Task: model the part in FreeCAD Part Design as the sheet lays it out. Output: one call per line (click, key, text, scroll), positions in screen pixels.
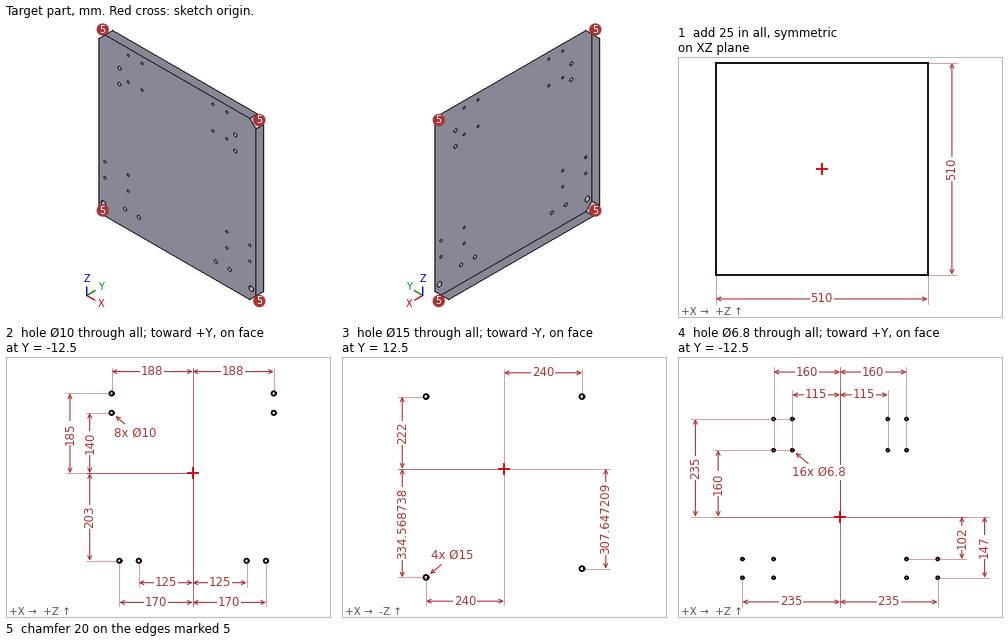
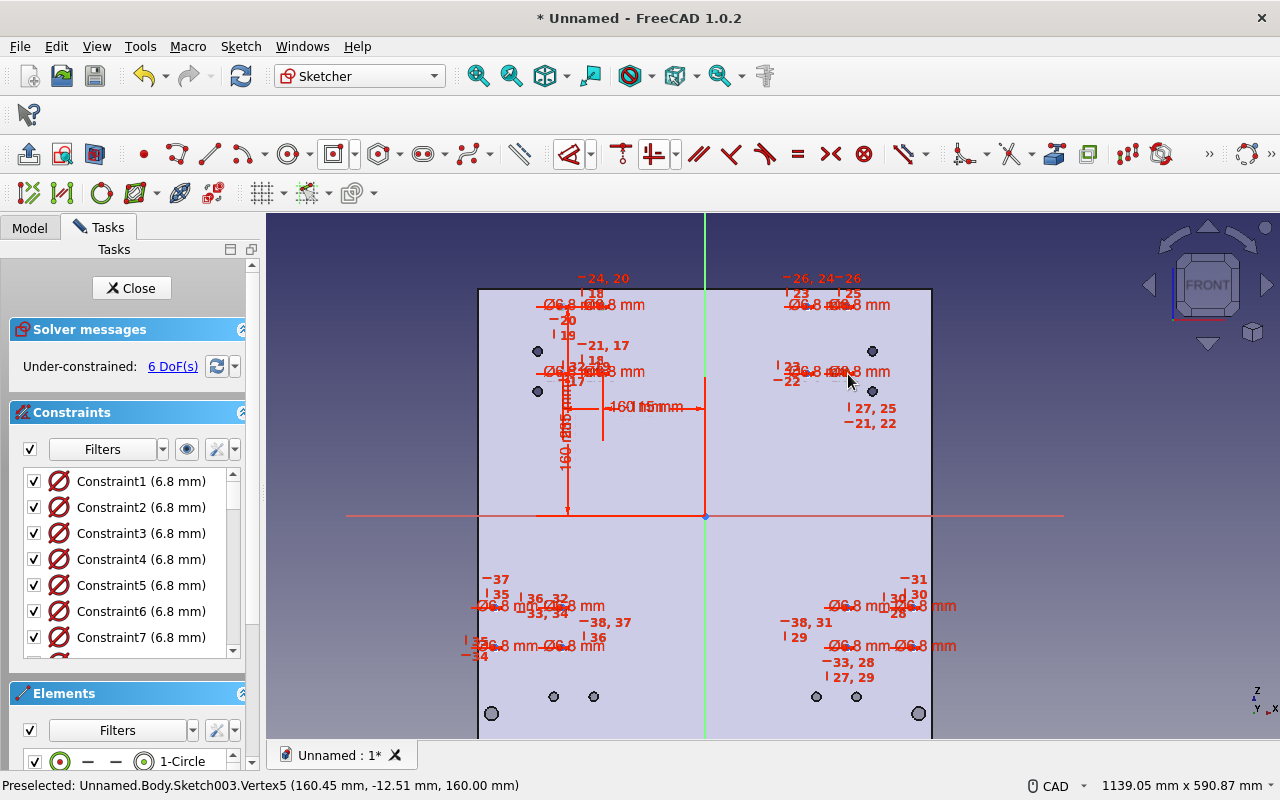
key(l)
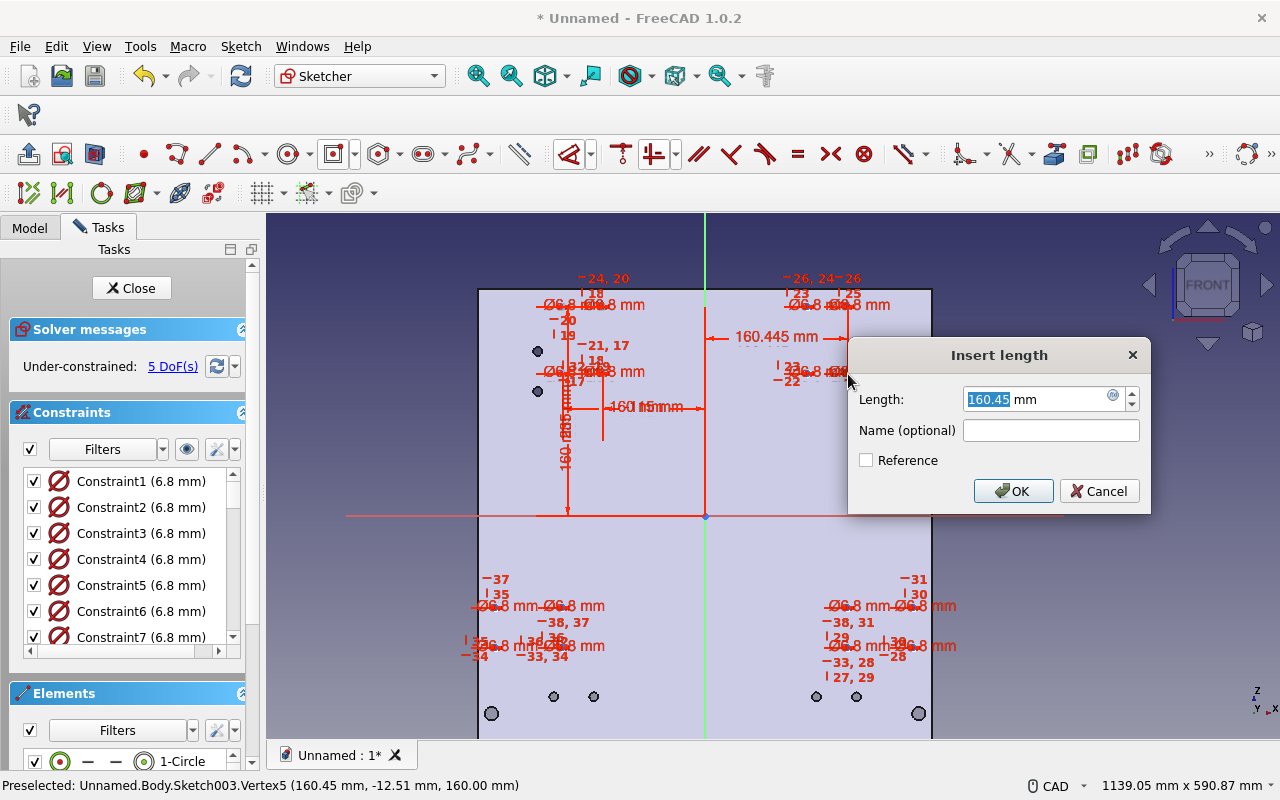
text(160)
key(Return)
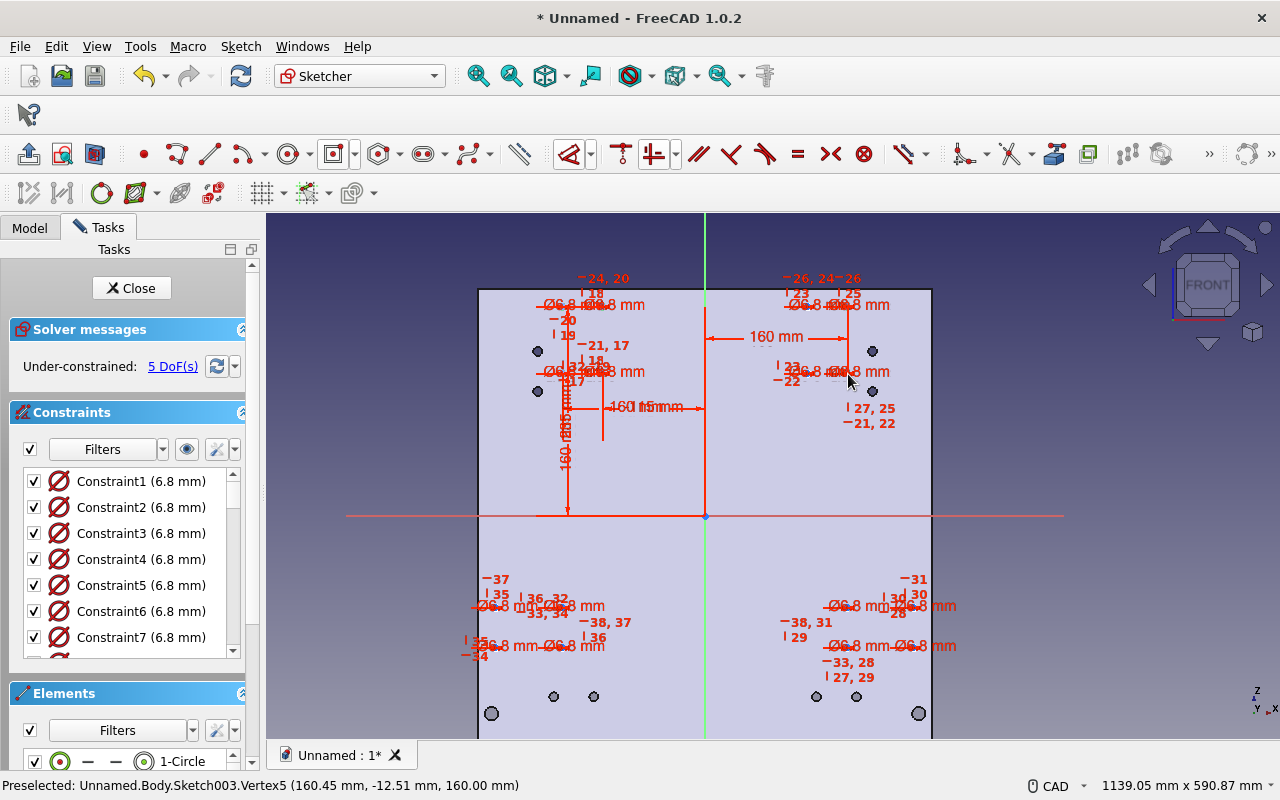
click(808, 374)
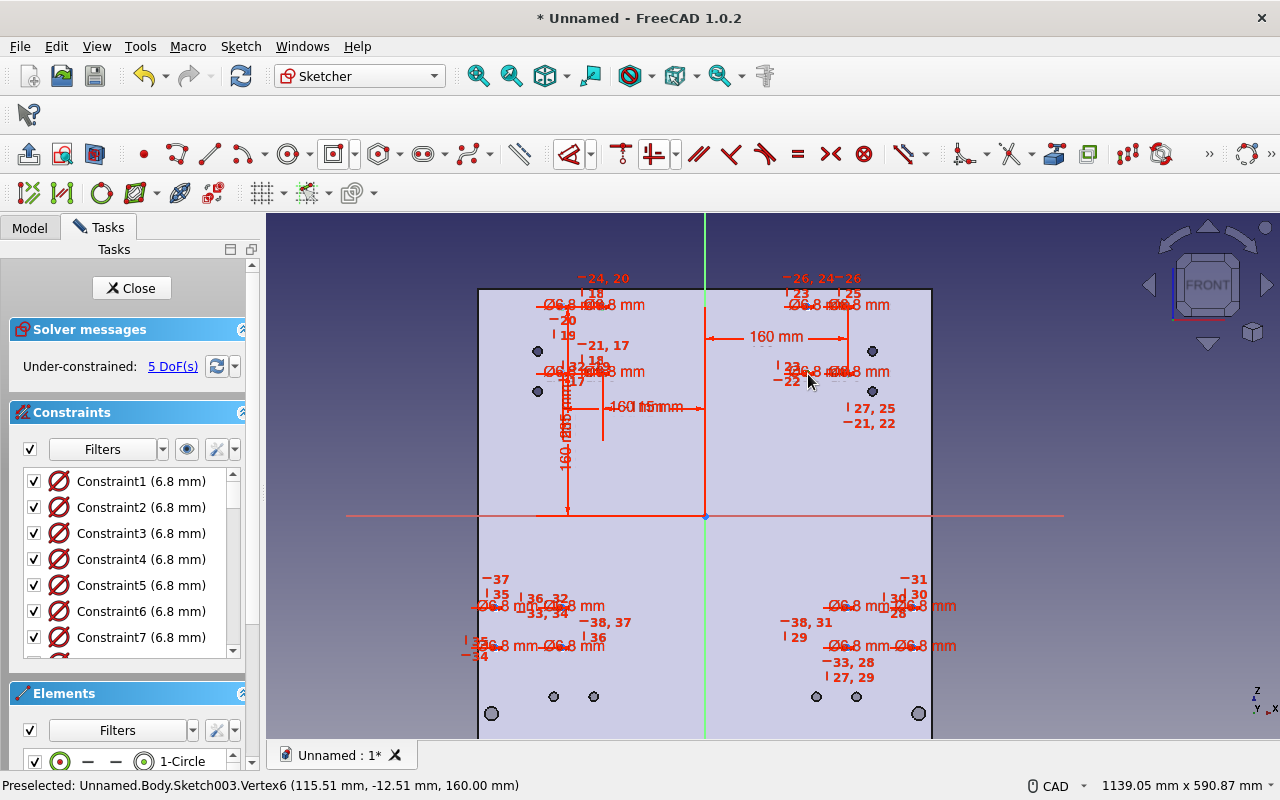
click(590, 154)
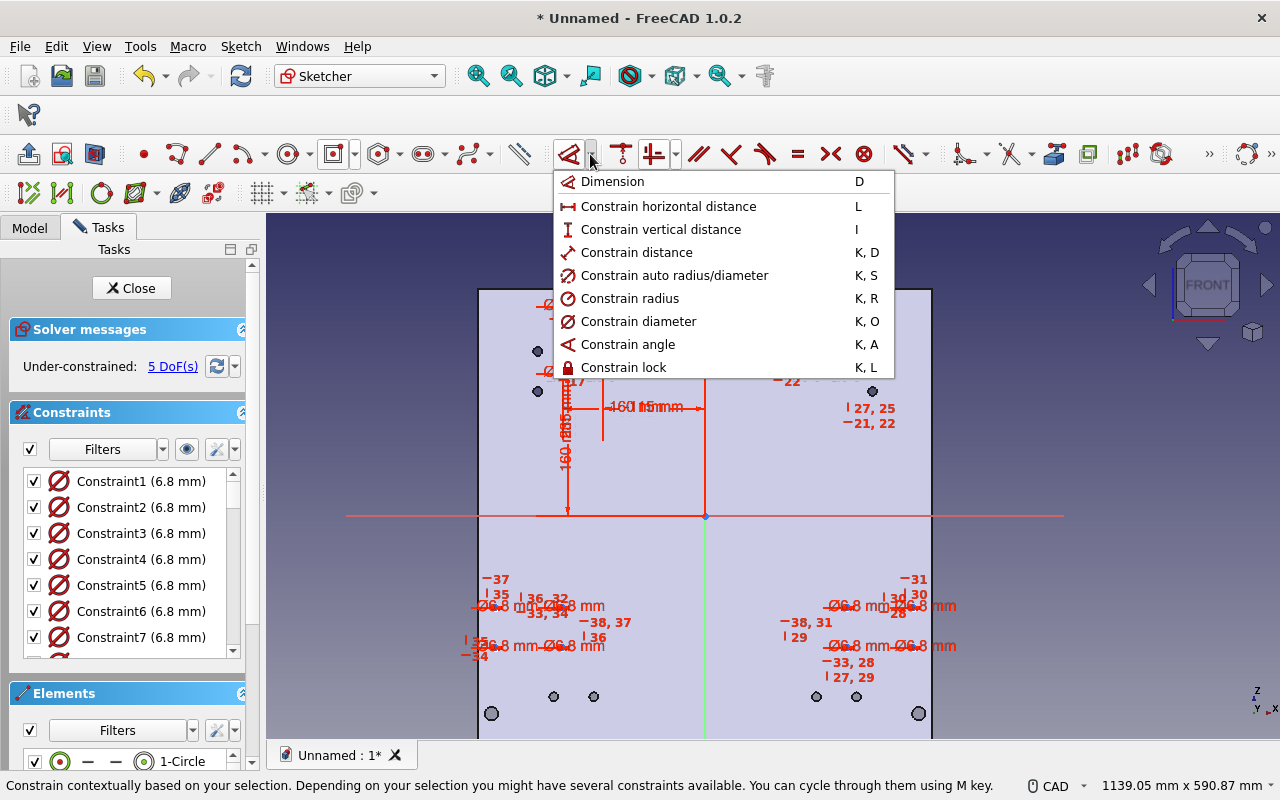
click(724, 206)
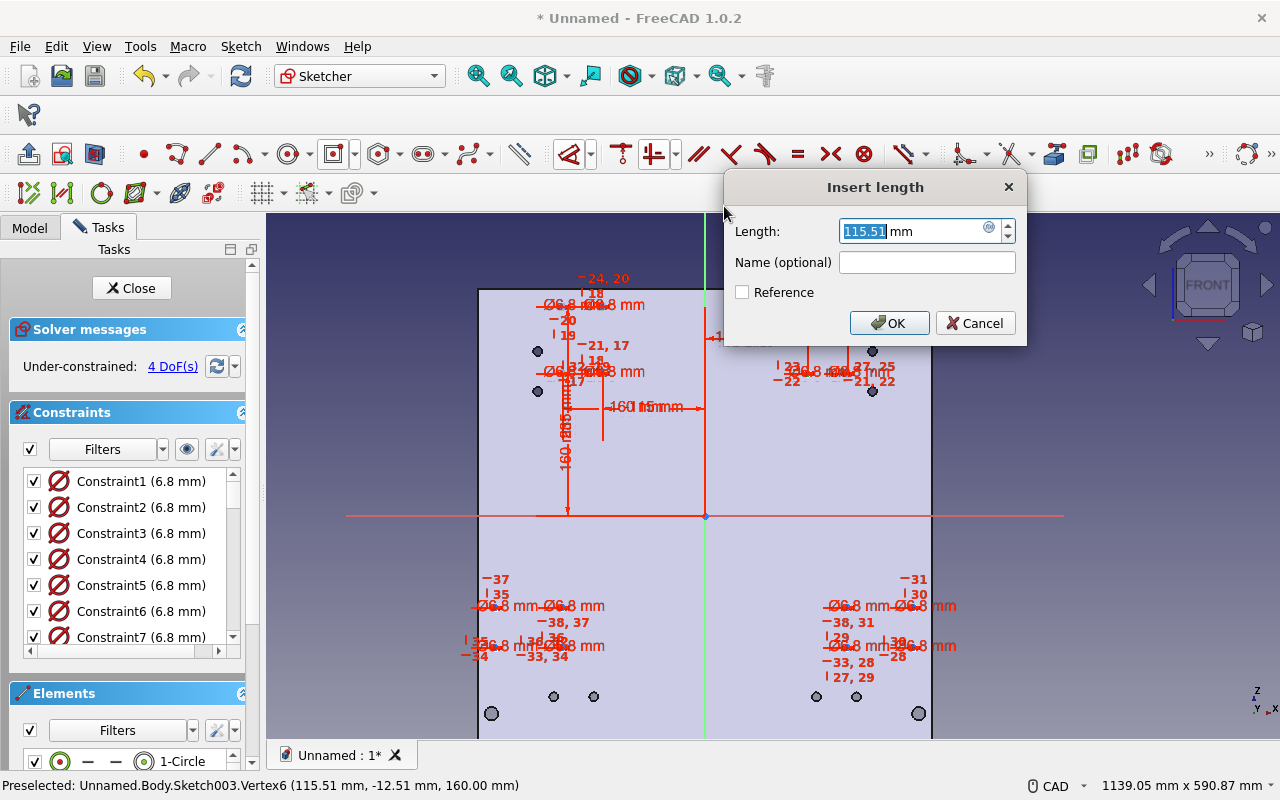
text(115)
key(Return)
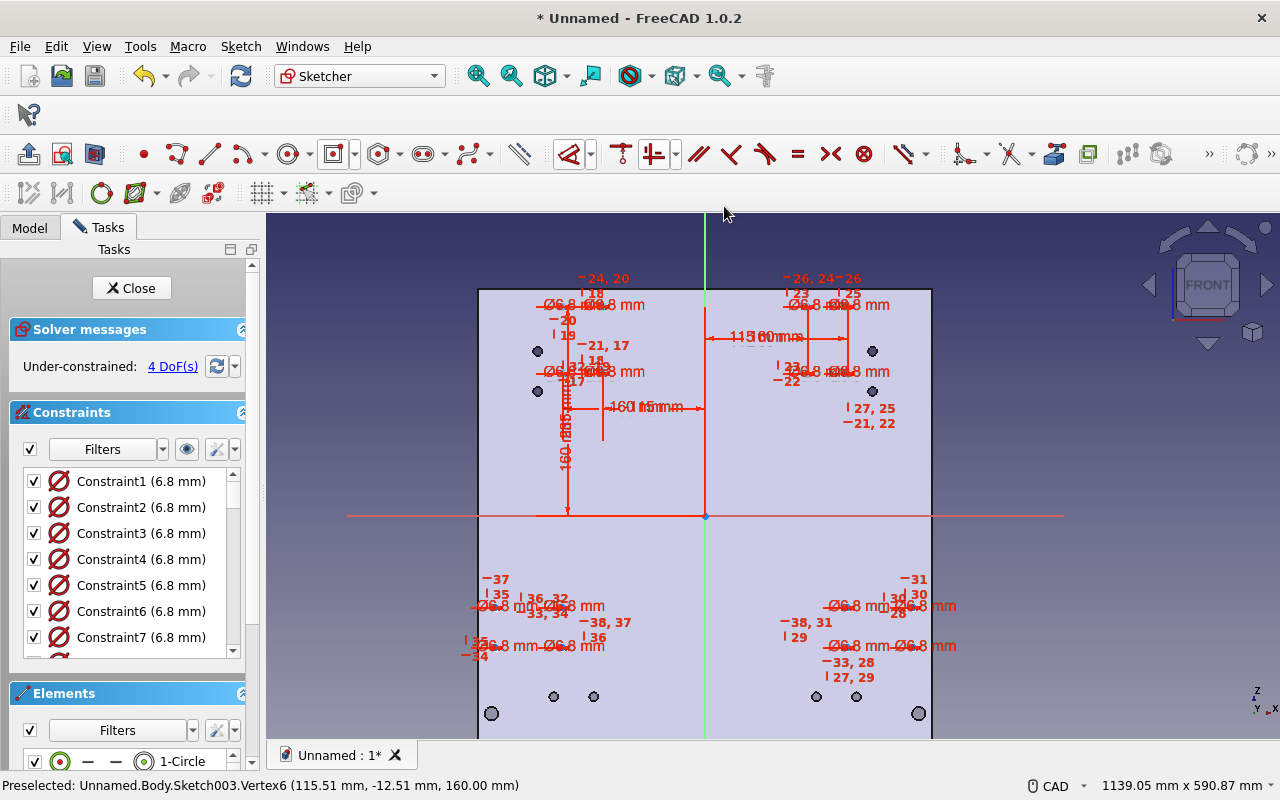
click(914, 648)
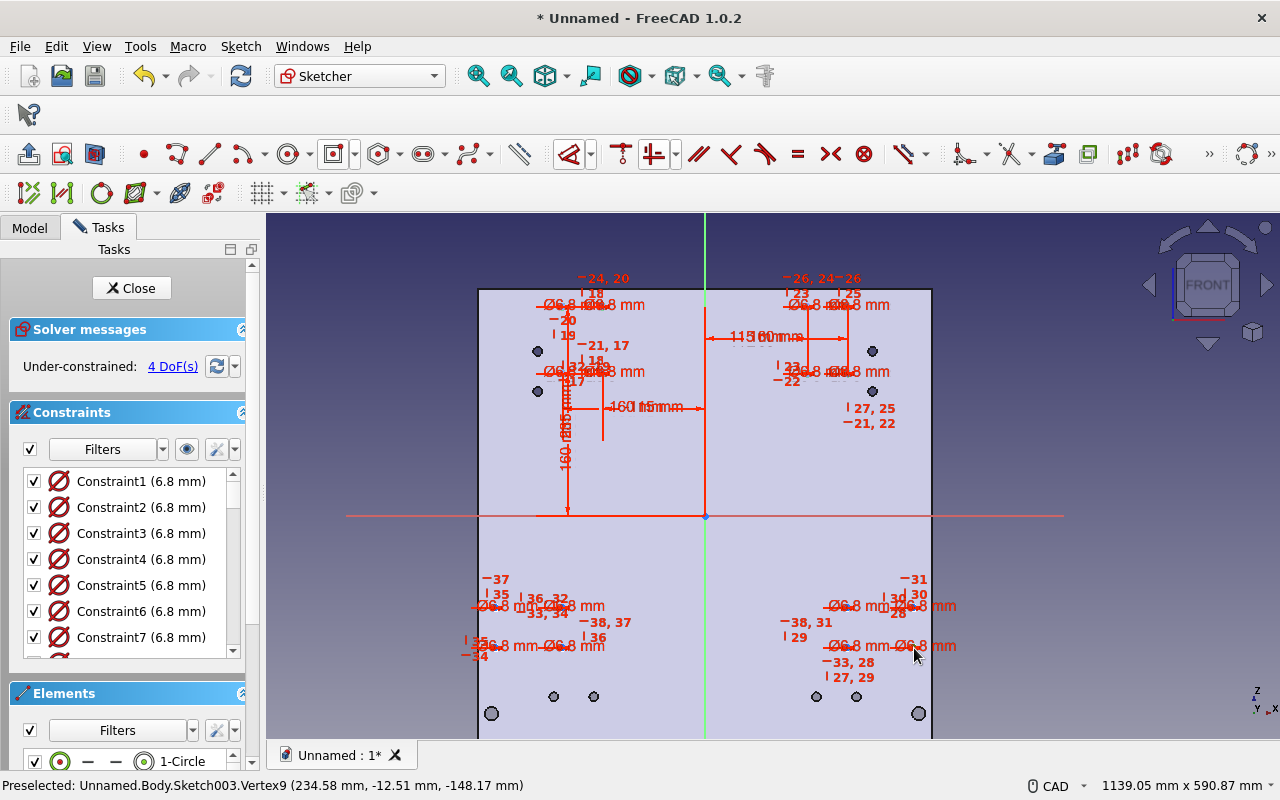
click(590, 154)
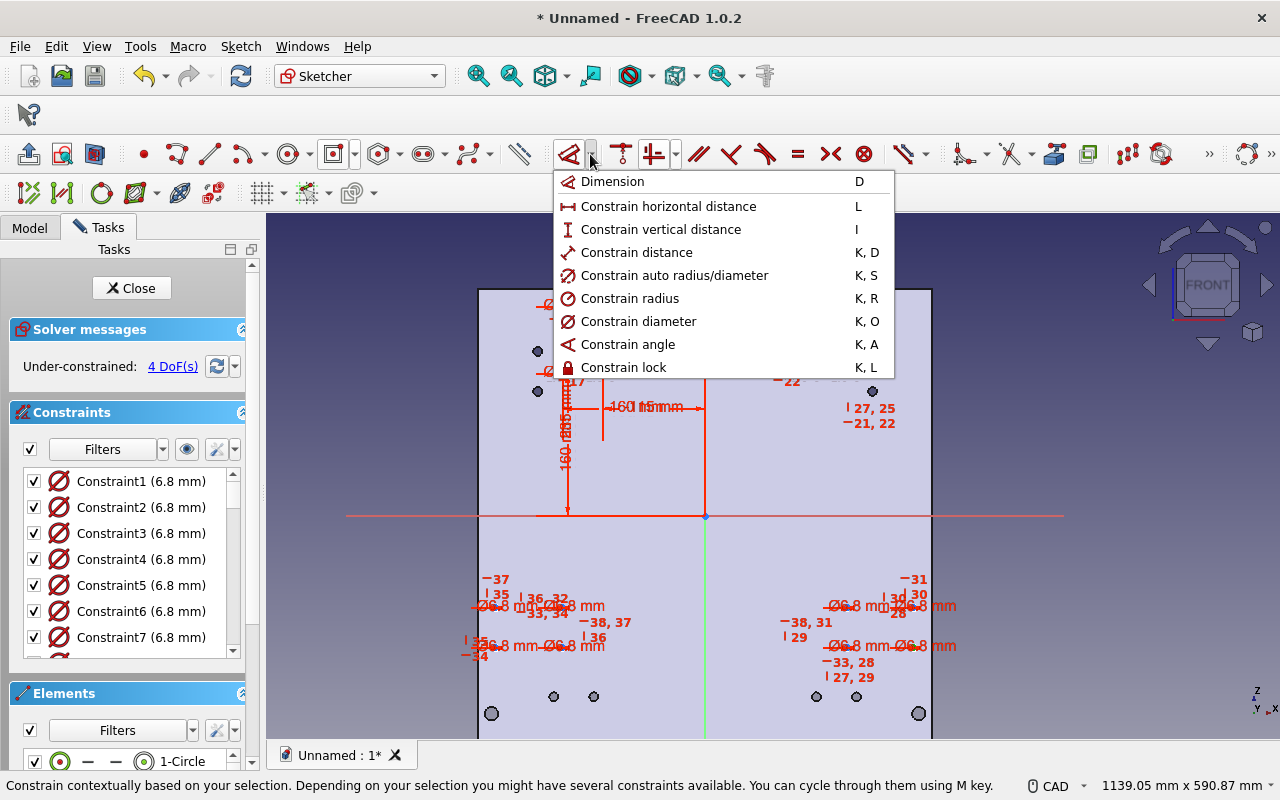
click(724, 206)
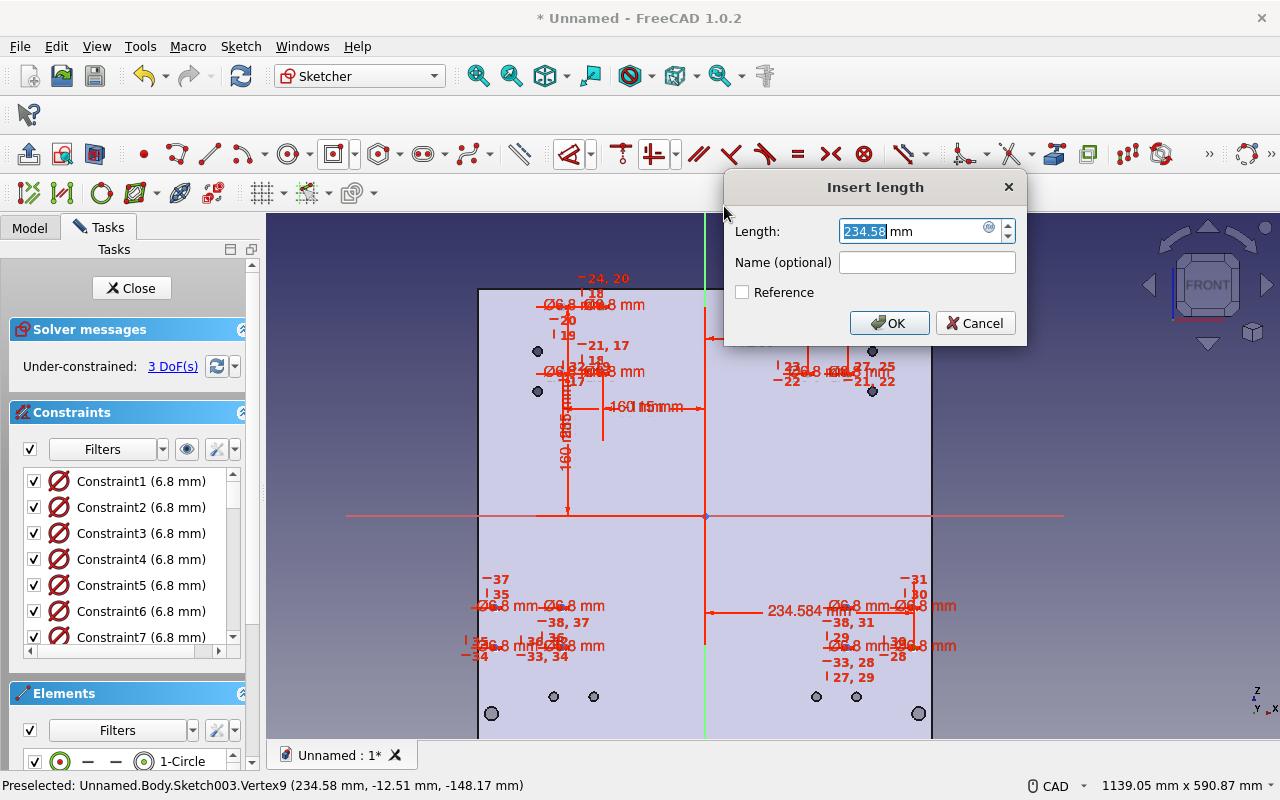
text(235)
key(Return)